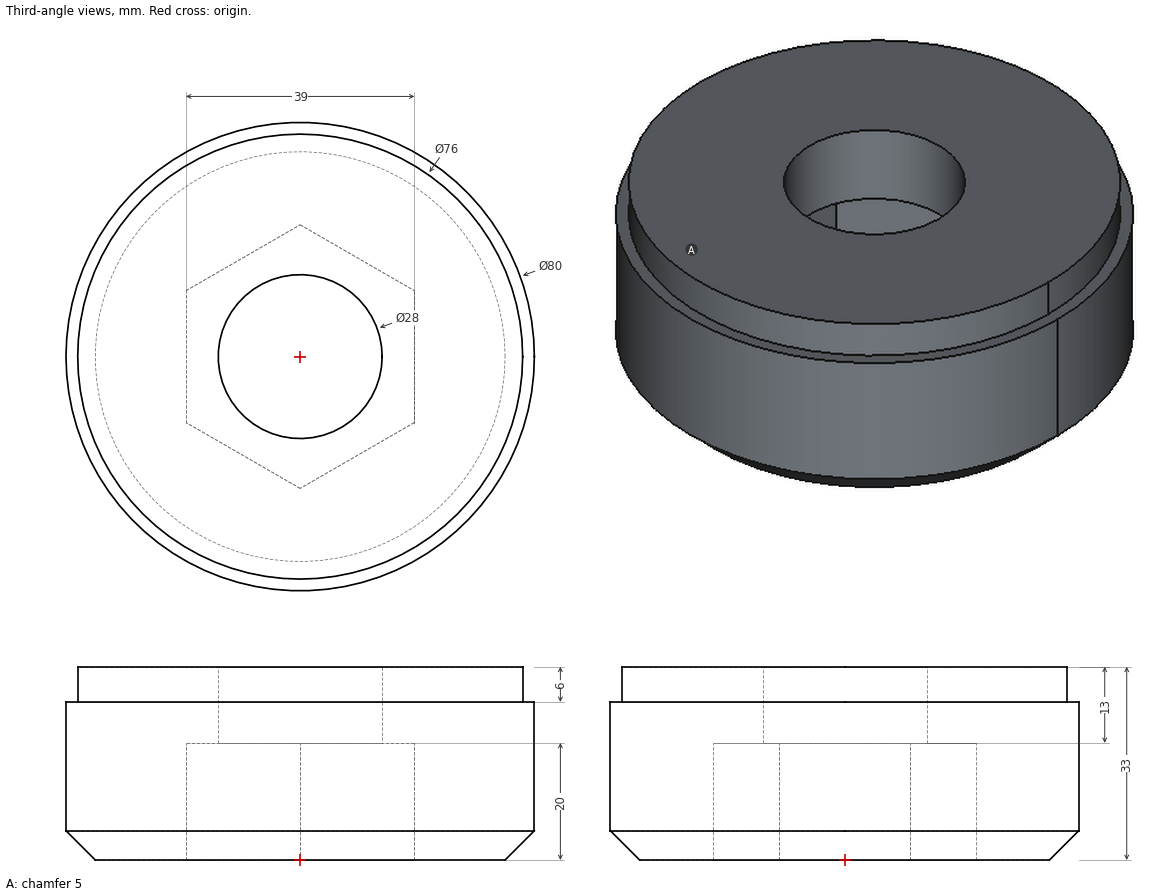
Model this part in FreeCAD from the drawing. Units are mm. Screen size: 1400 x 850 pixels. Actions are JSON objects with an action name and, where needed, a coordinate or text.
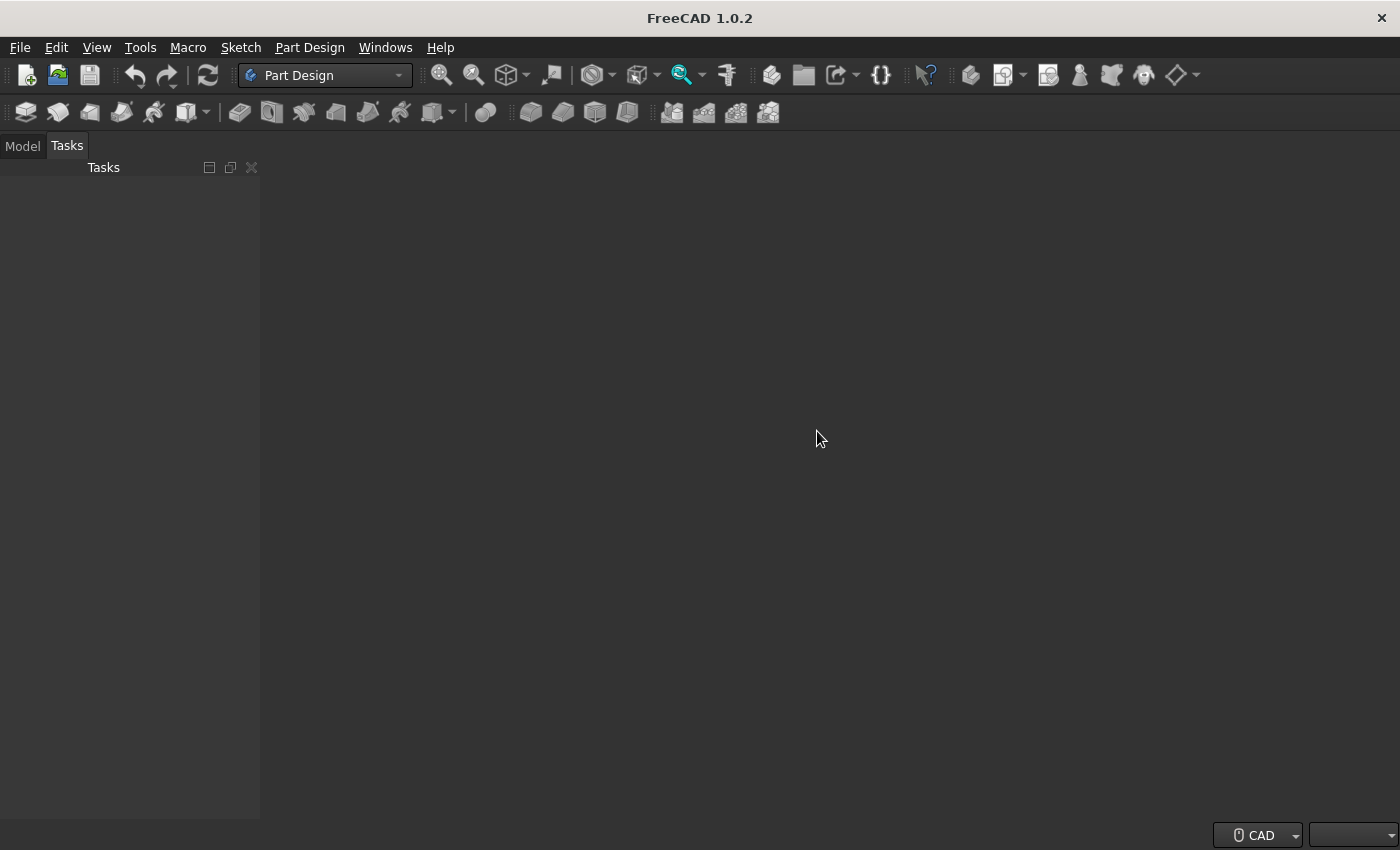
{"action": "left_click", "coordinate": [26, 76]}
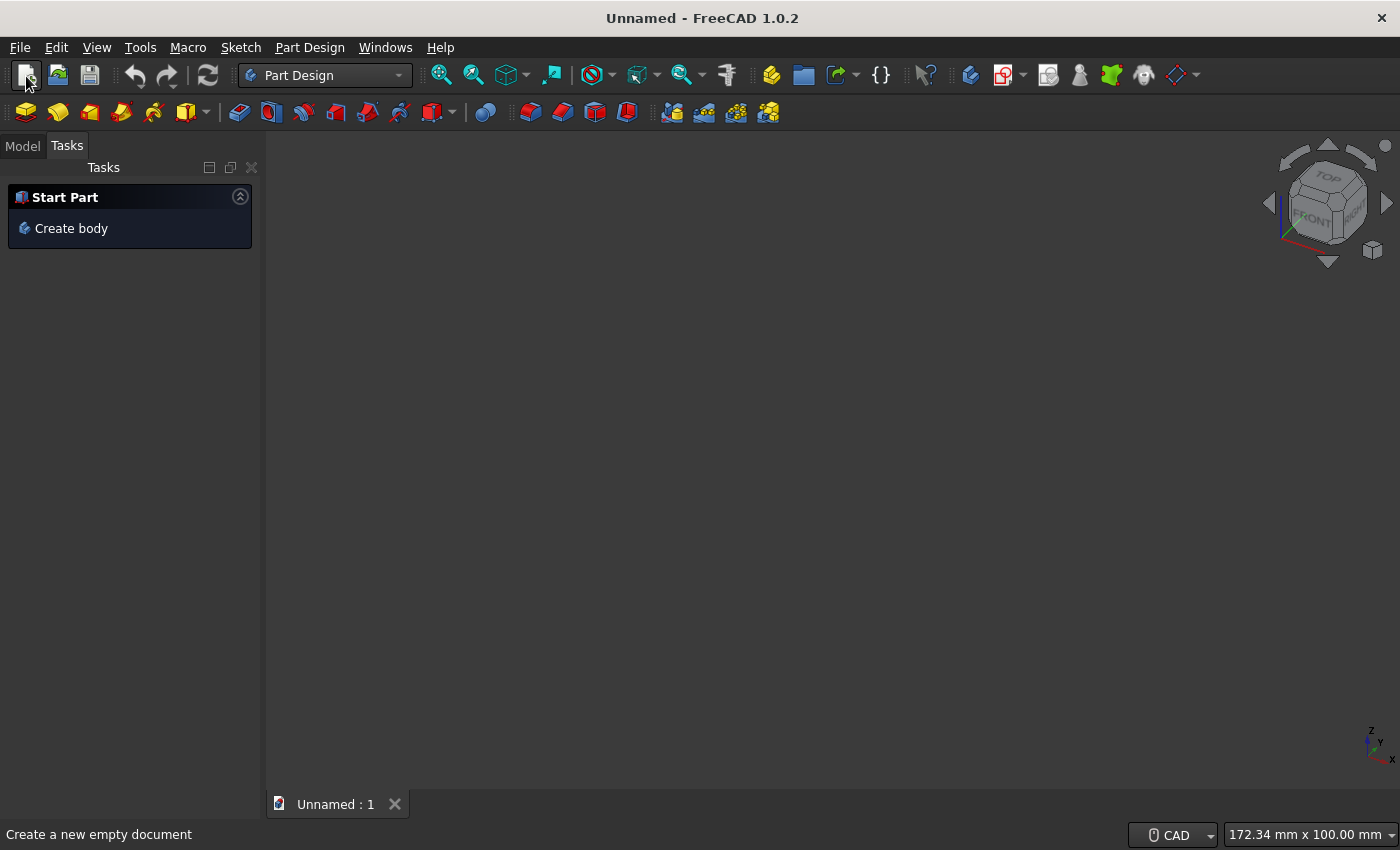
{"action": "left_click", "coordinate": [1004, 76]}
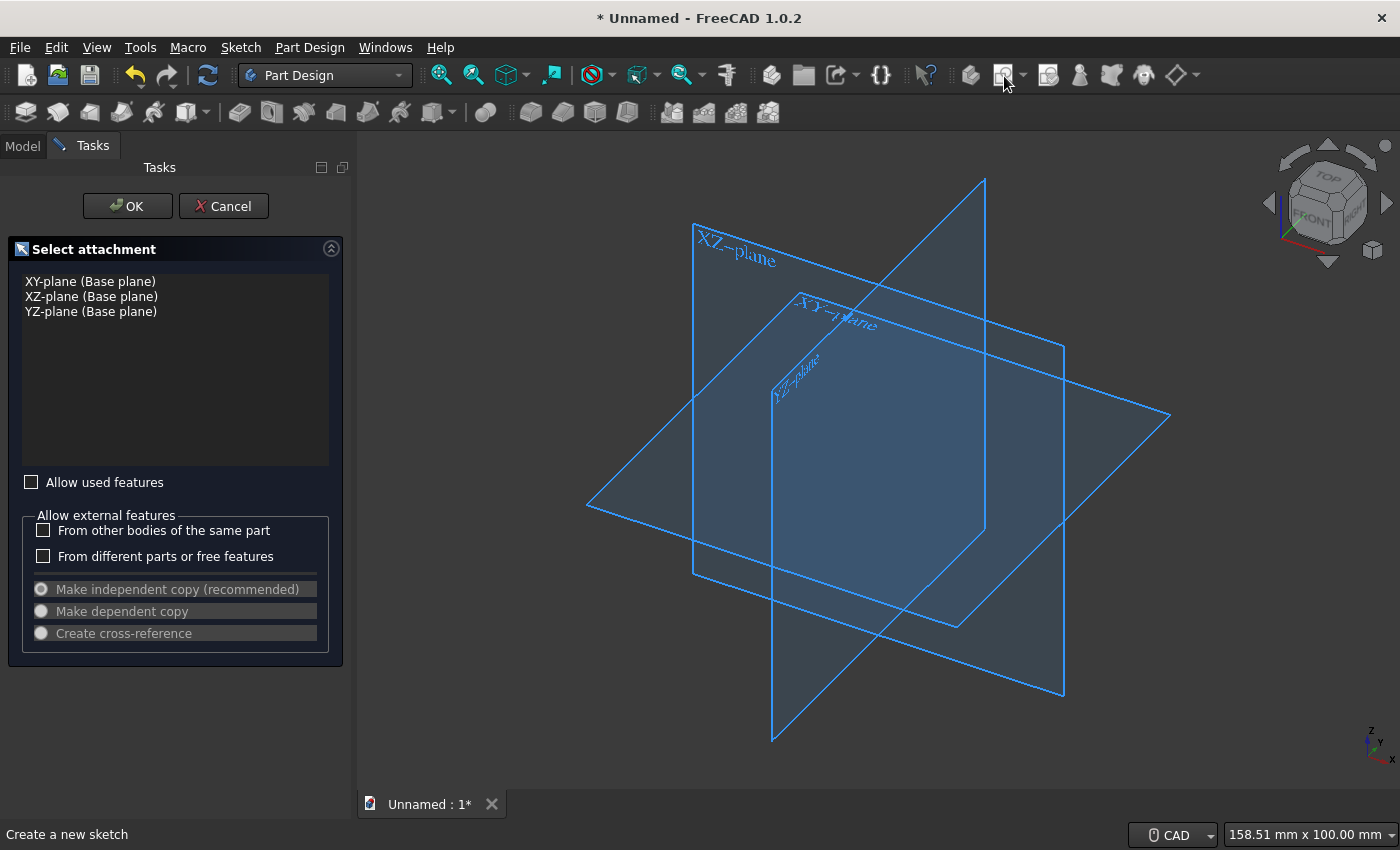
{"action": "left_click", "coordinate": [82, 282]}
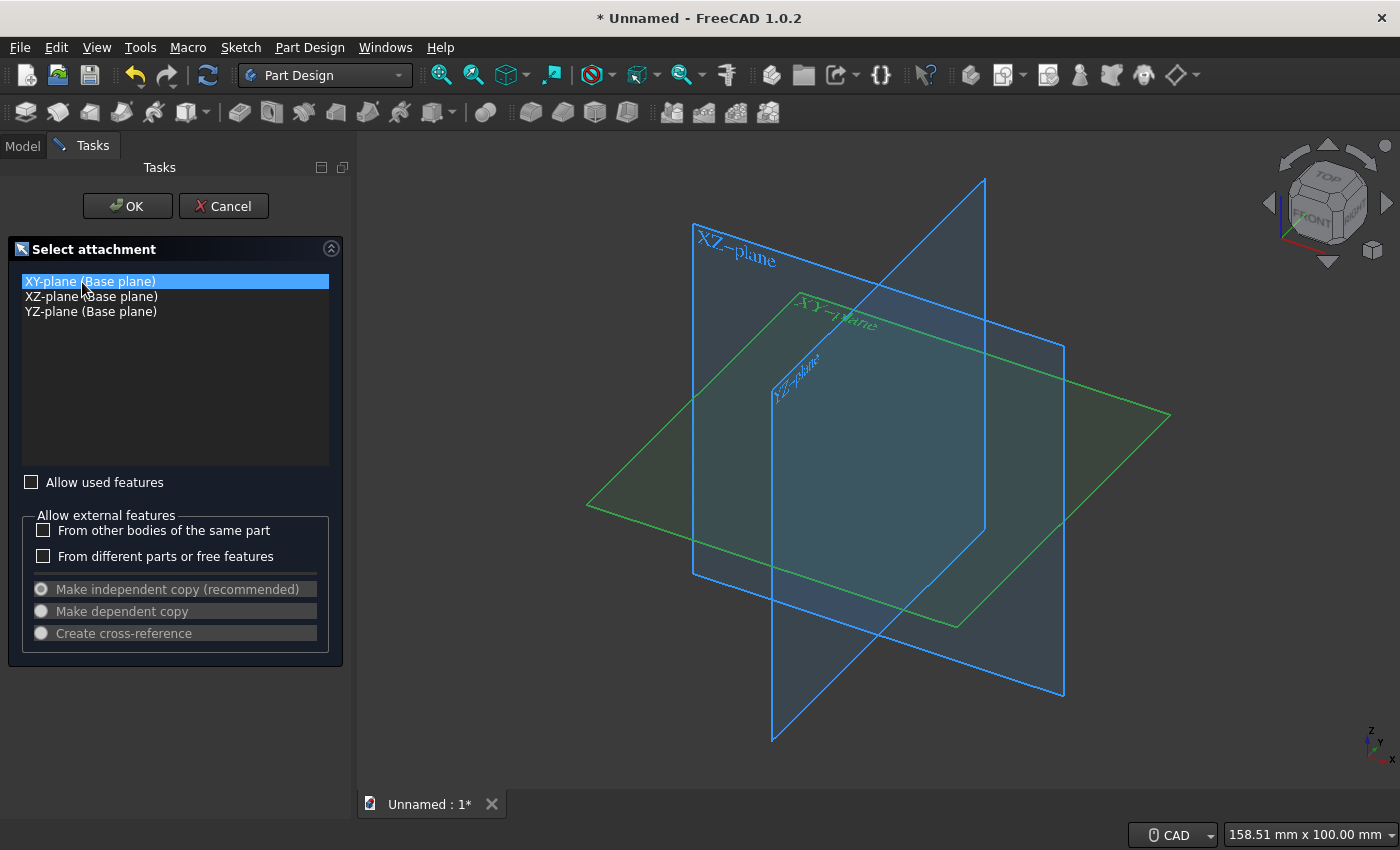
{"action": "left_click", "coordinate": [128, 206]}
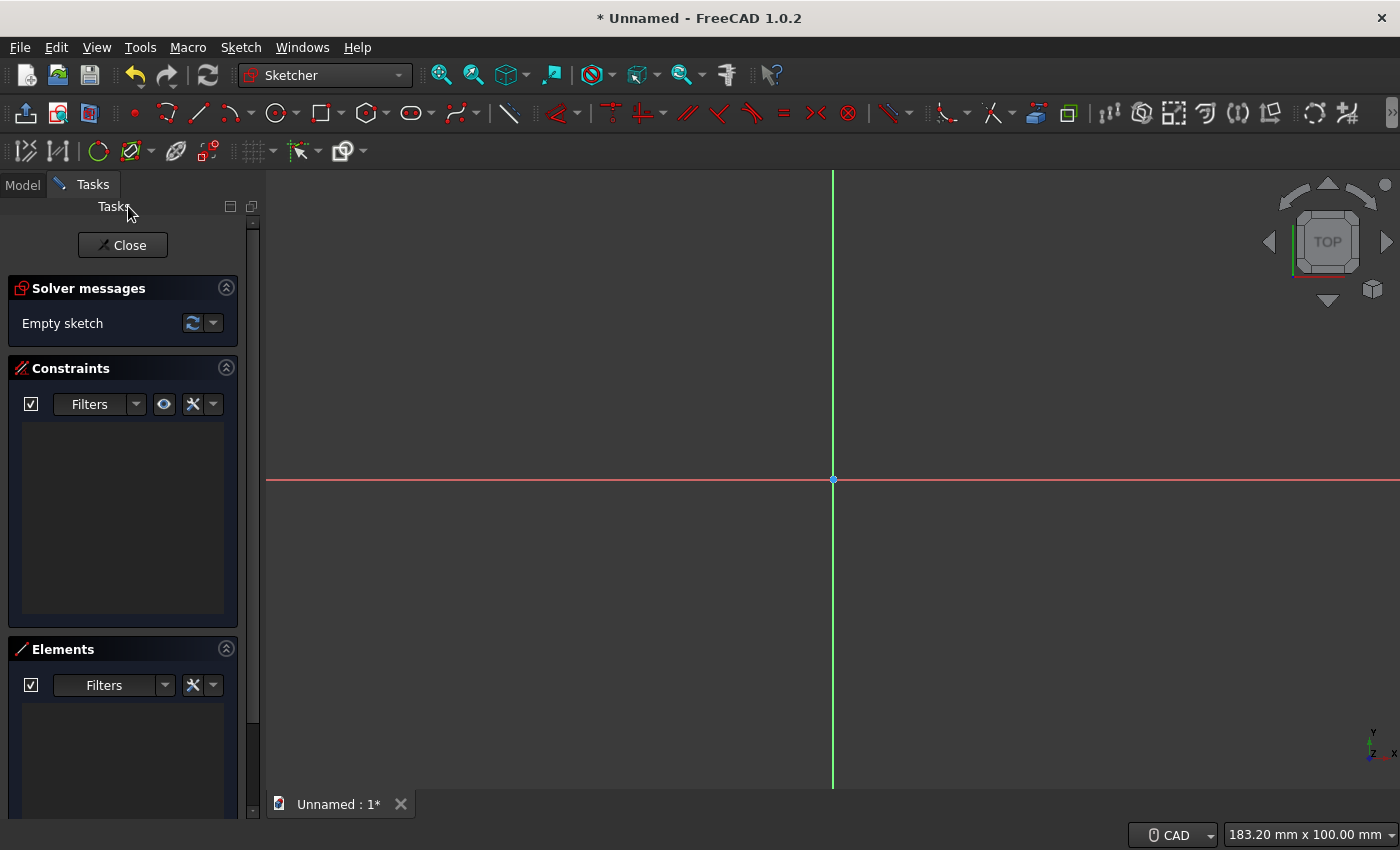
{"action": "left_click", "coordinate": [276, 114]}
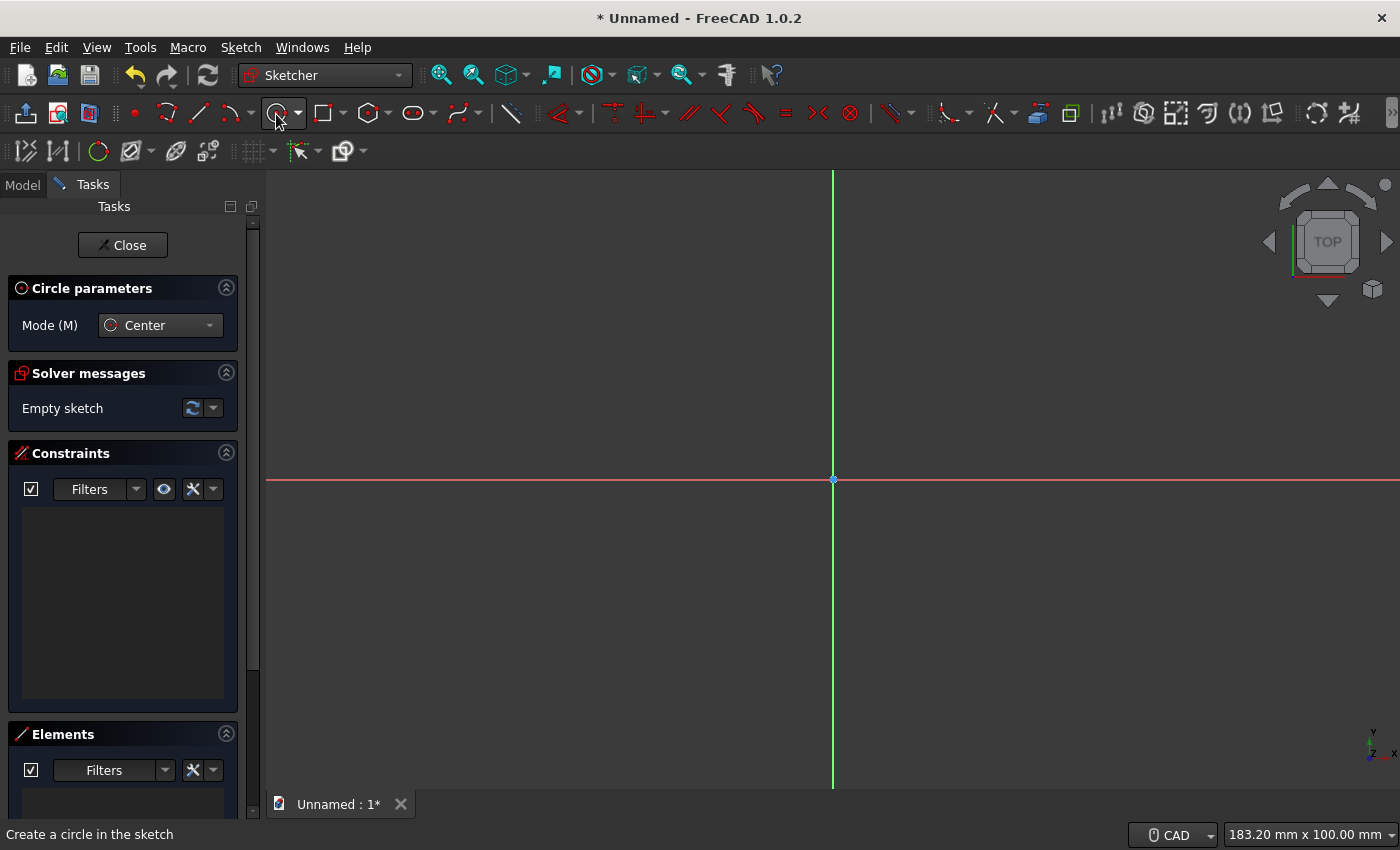
{"action": "left_click", "coordinate": [833, 480]}
{"action": "left_click", "coordinate": [1008, 304]}
{"action": "key", "text": "Escape"}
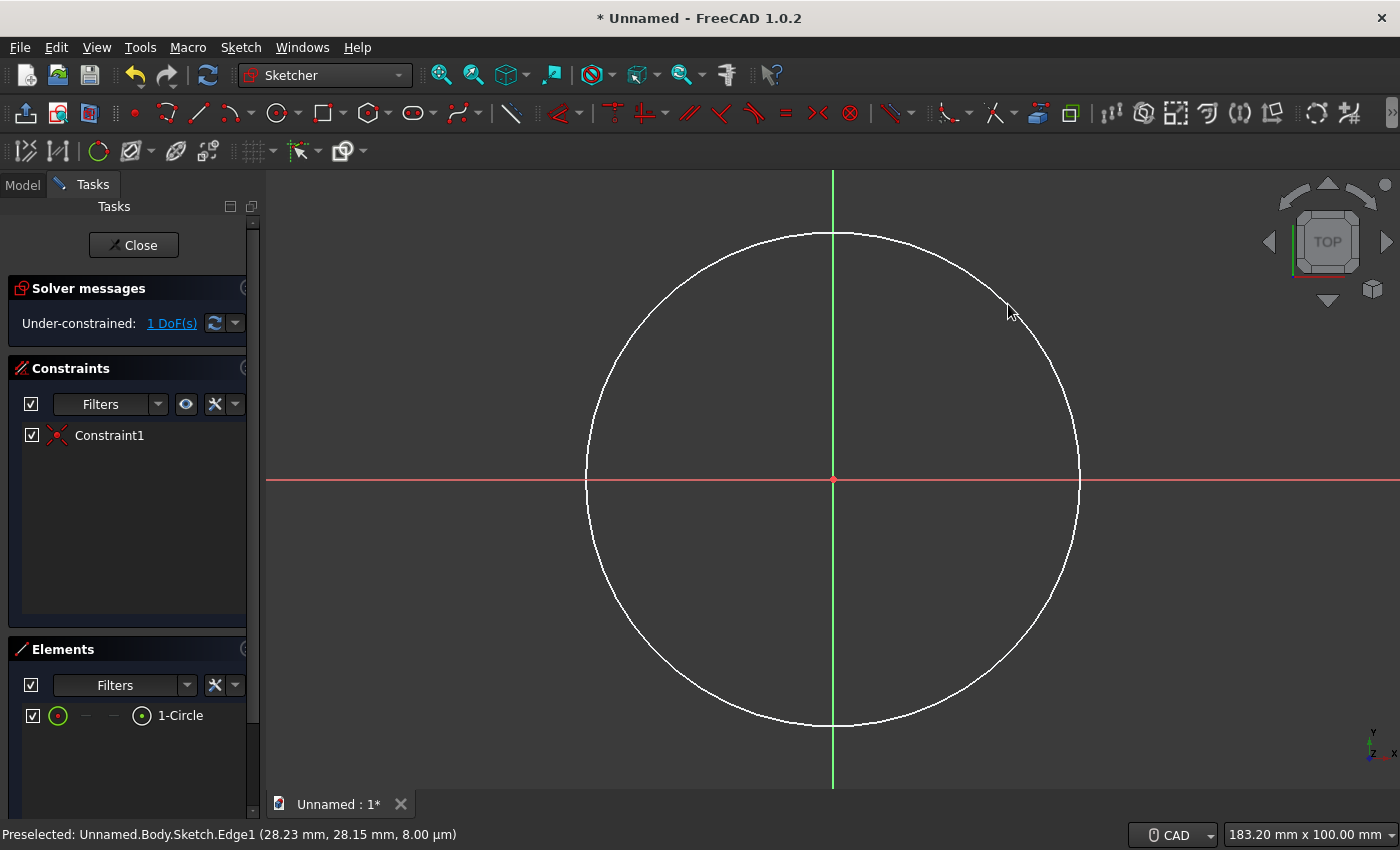
{"action": "left_click", "coordinate": [558, 114]}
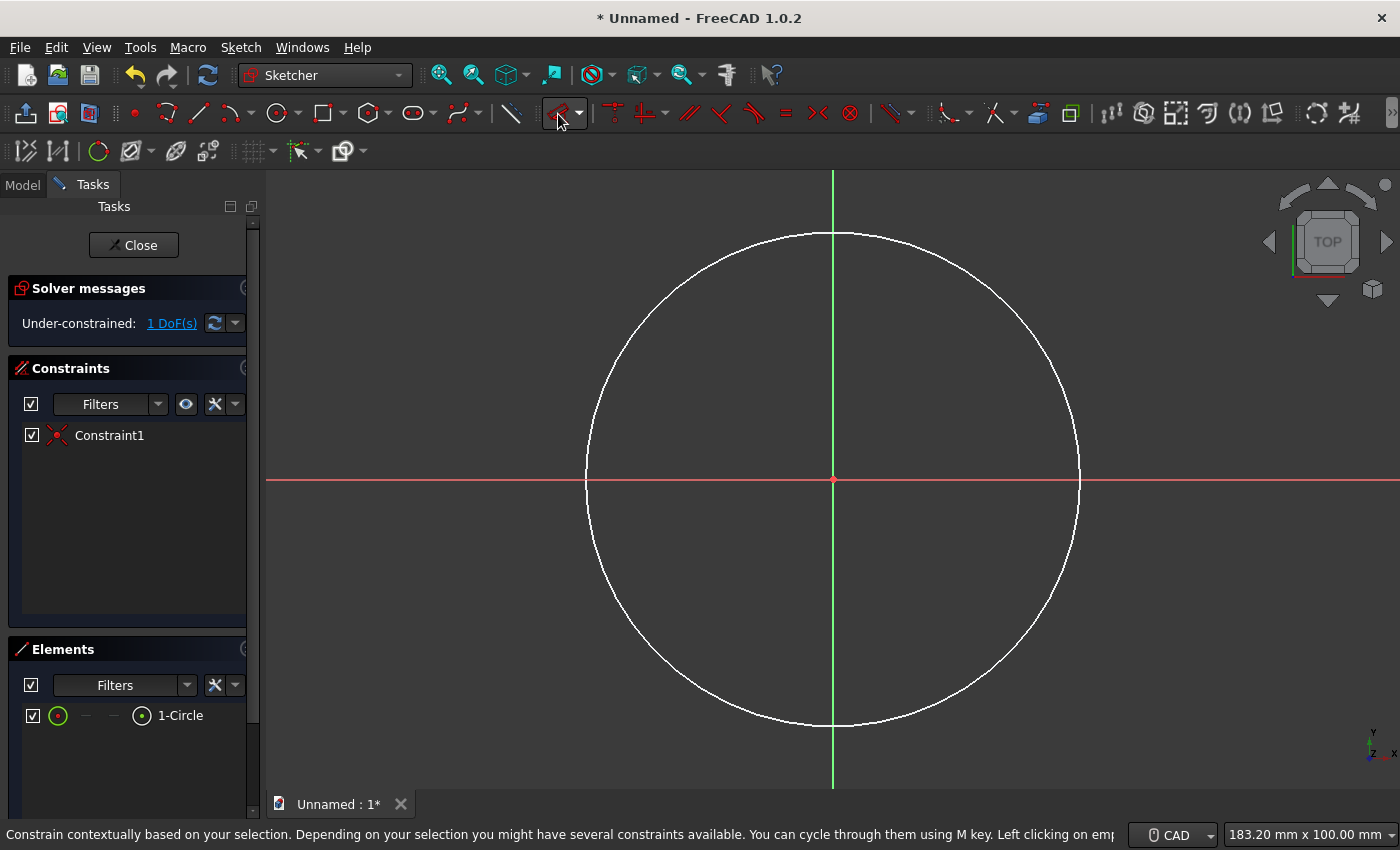
{"action": "left_click", "coordinate": [1007, 304]}
{"action": "left_click", "coordinate": [1030, 281]}